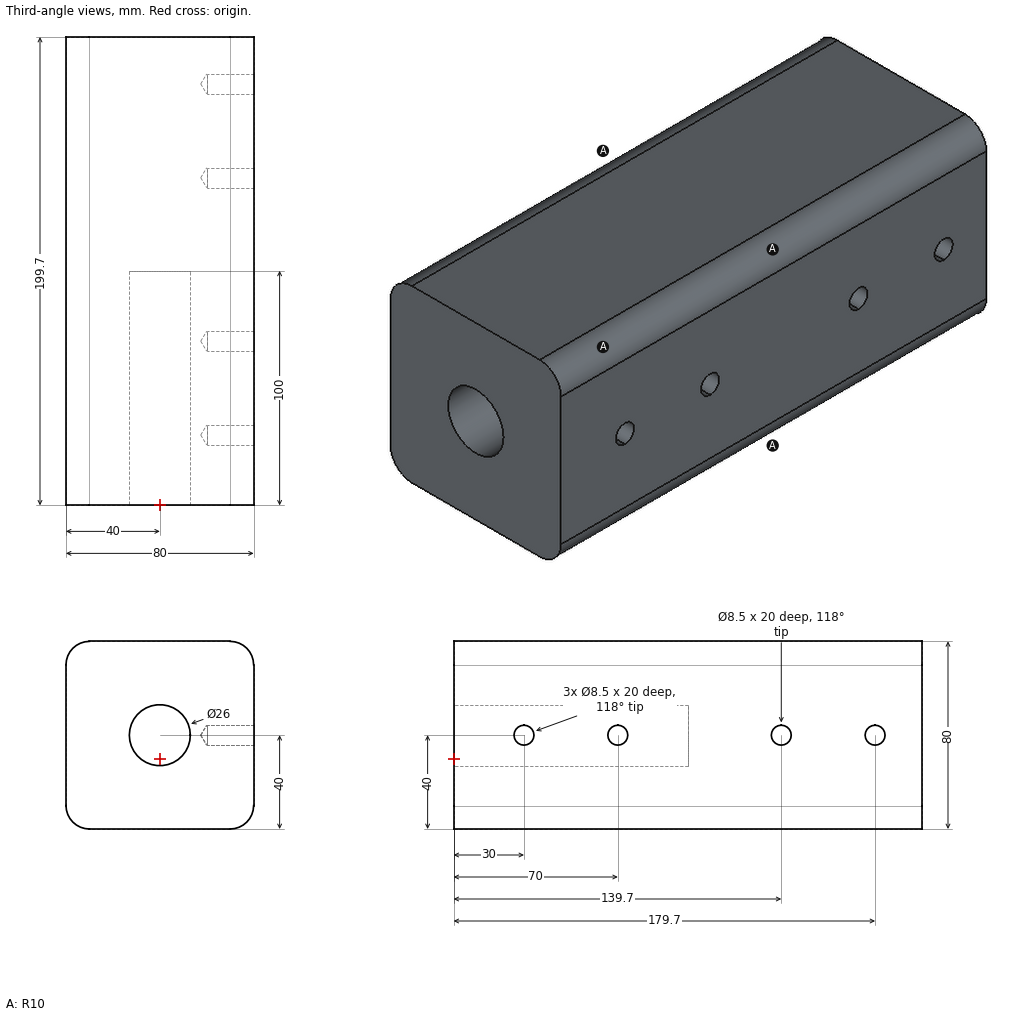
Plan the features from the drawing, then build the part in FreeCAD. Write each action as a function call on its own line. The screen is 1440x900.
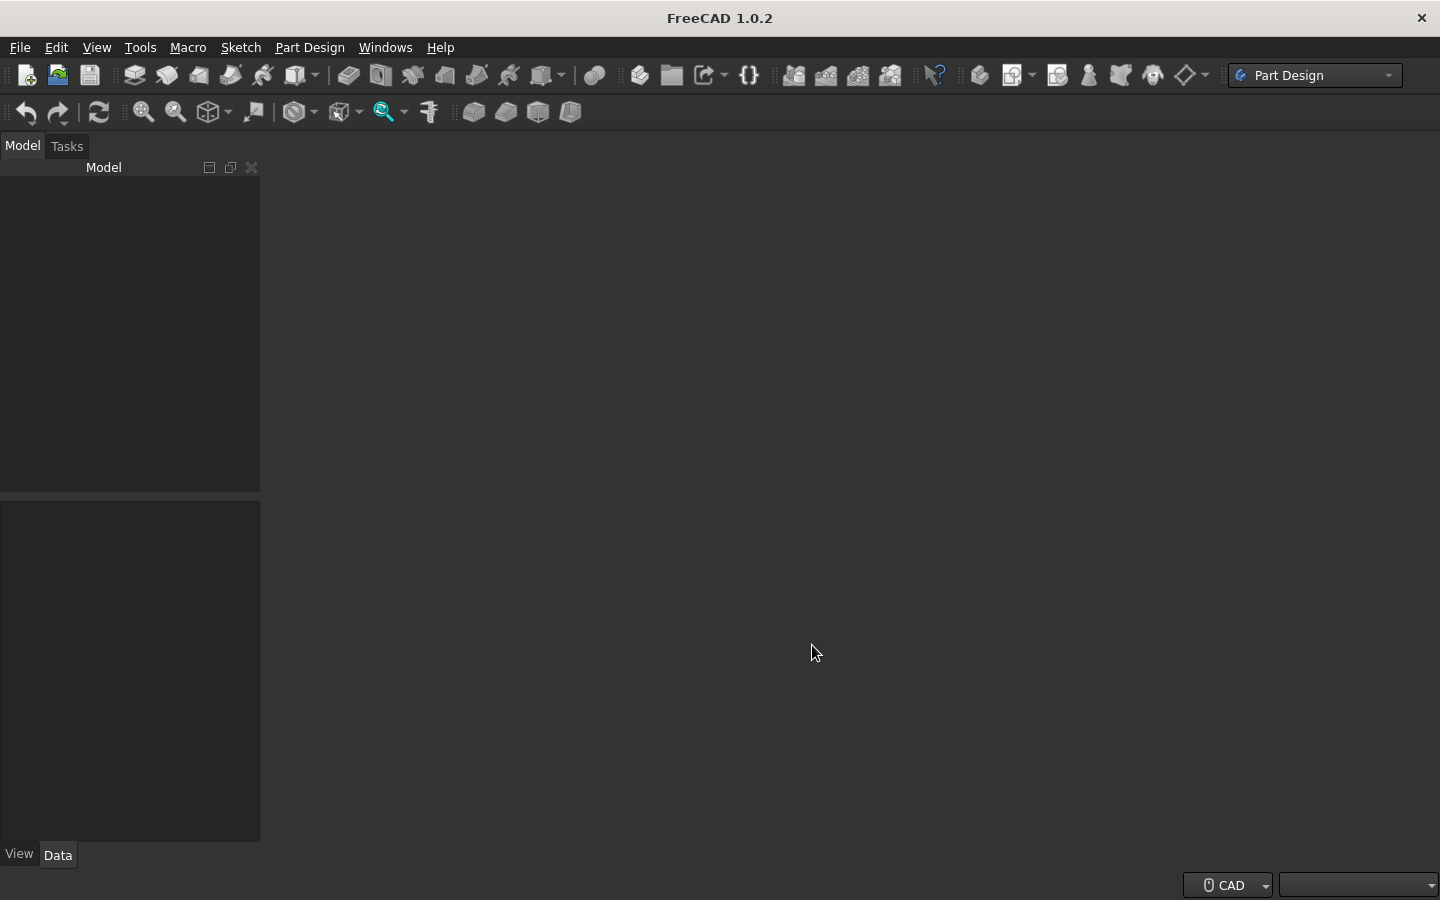
click(26, 76)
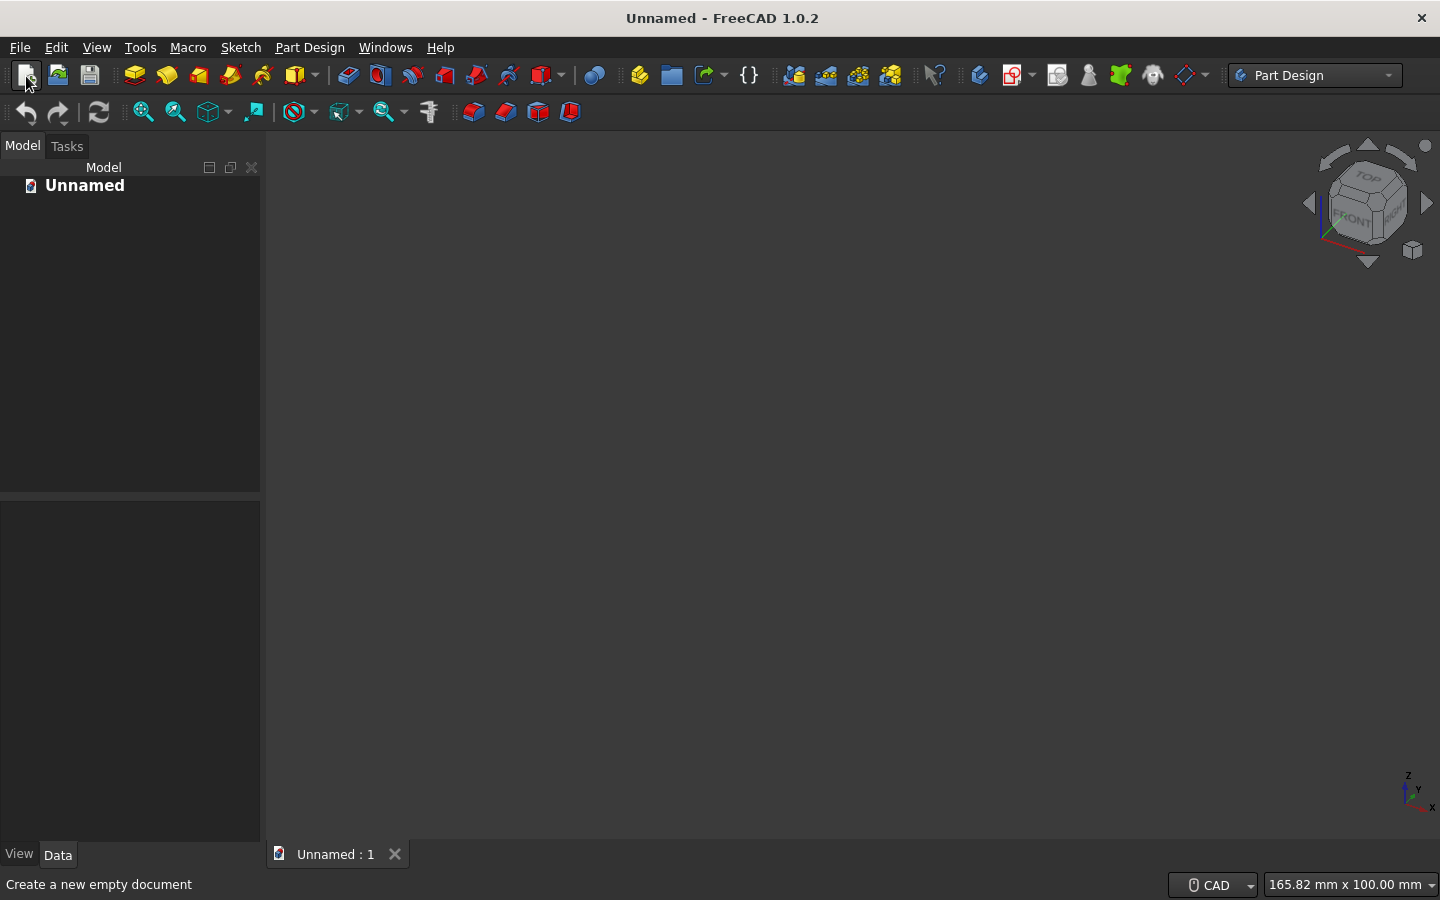
click(980, 76)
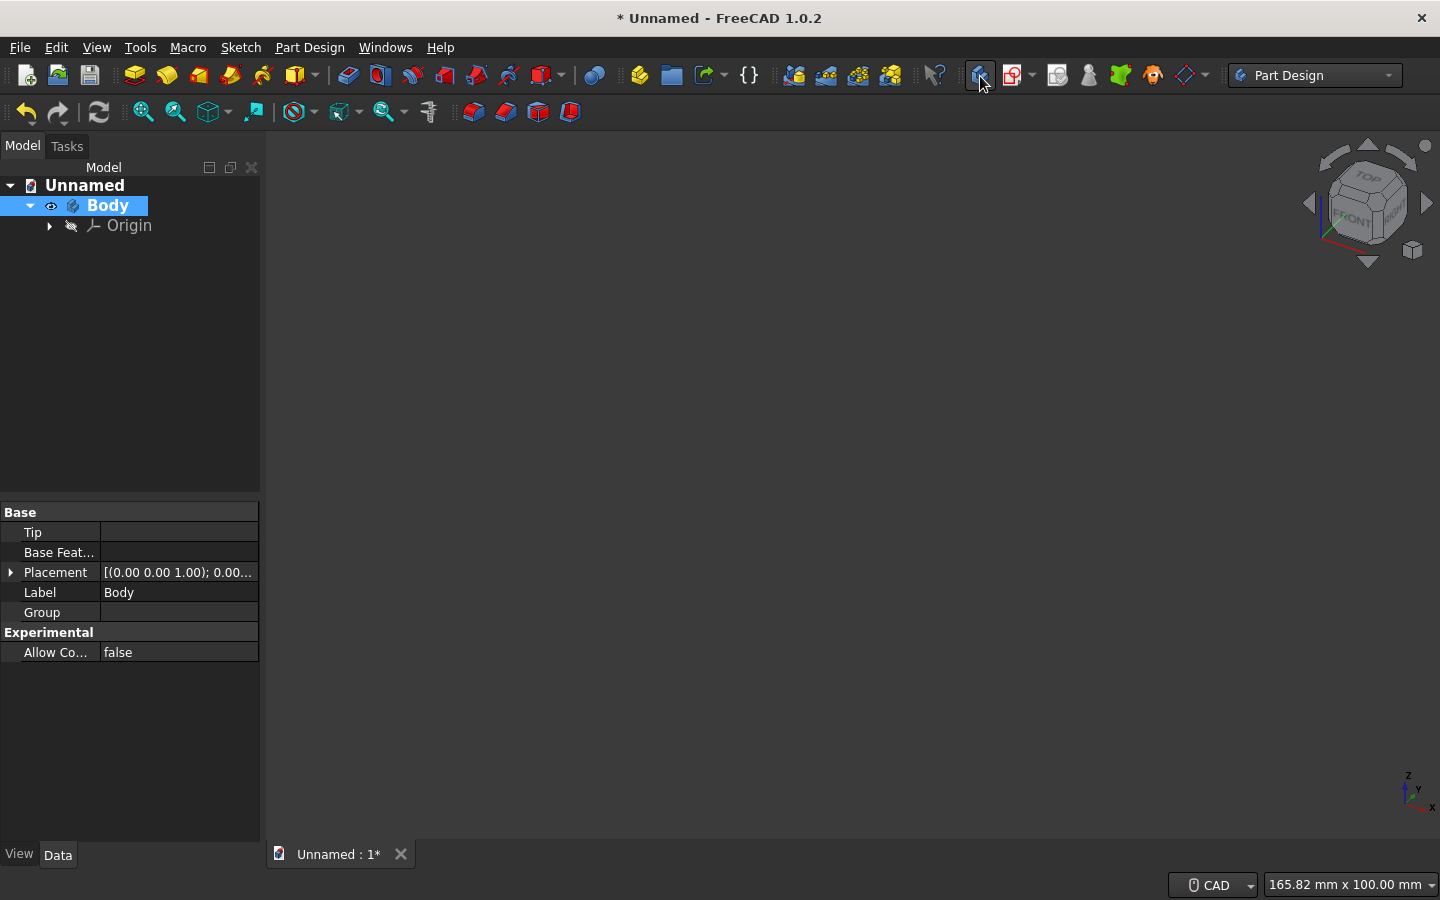
click(50, 226)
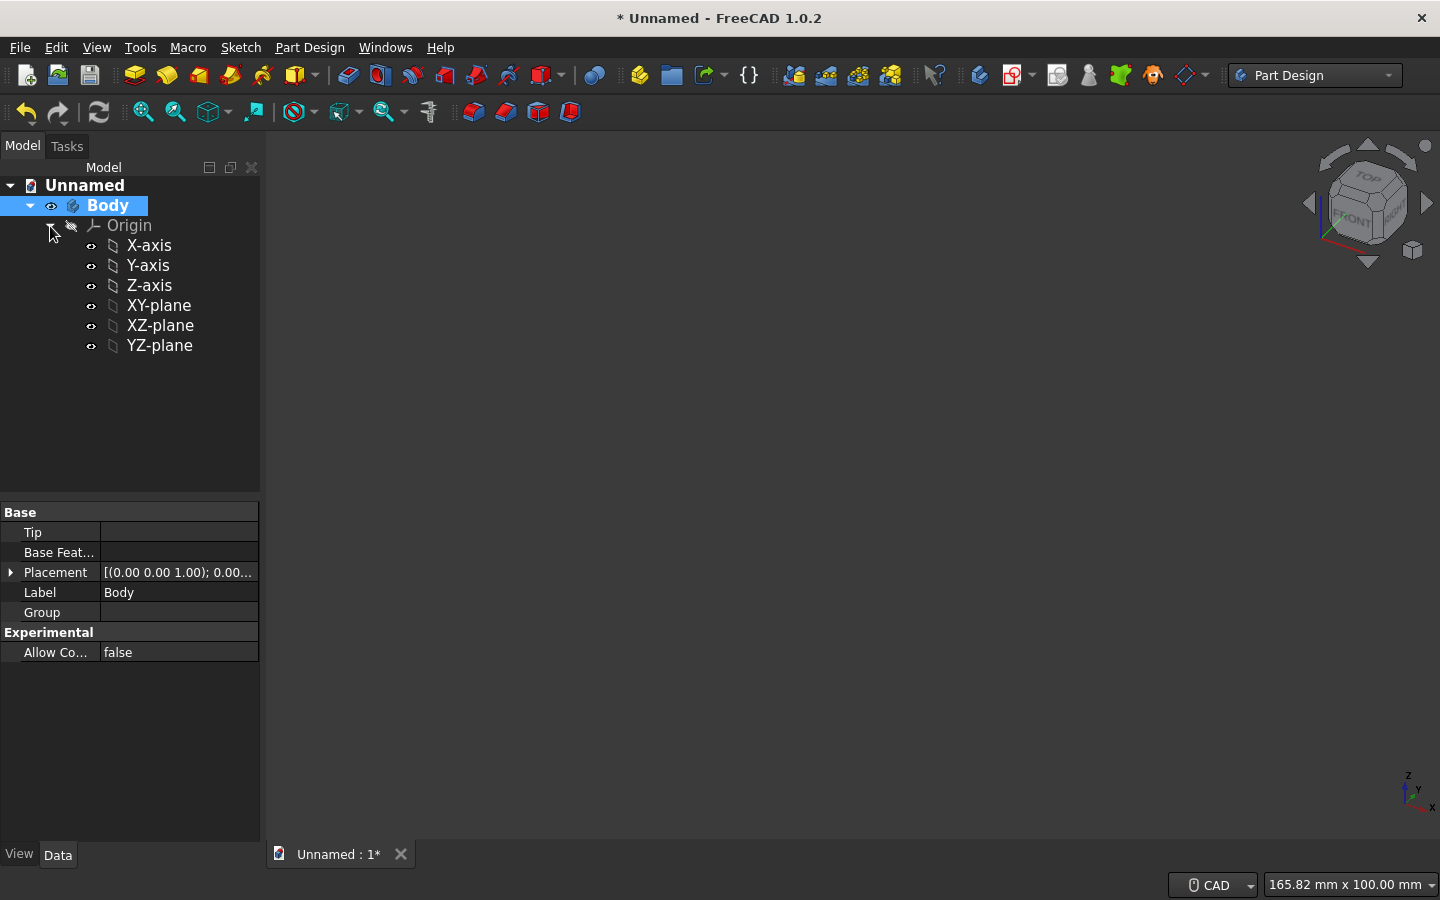
click(136, 306)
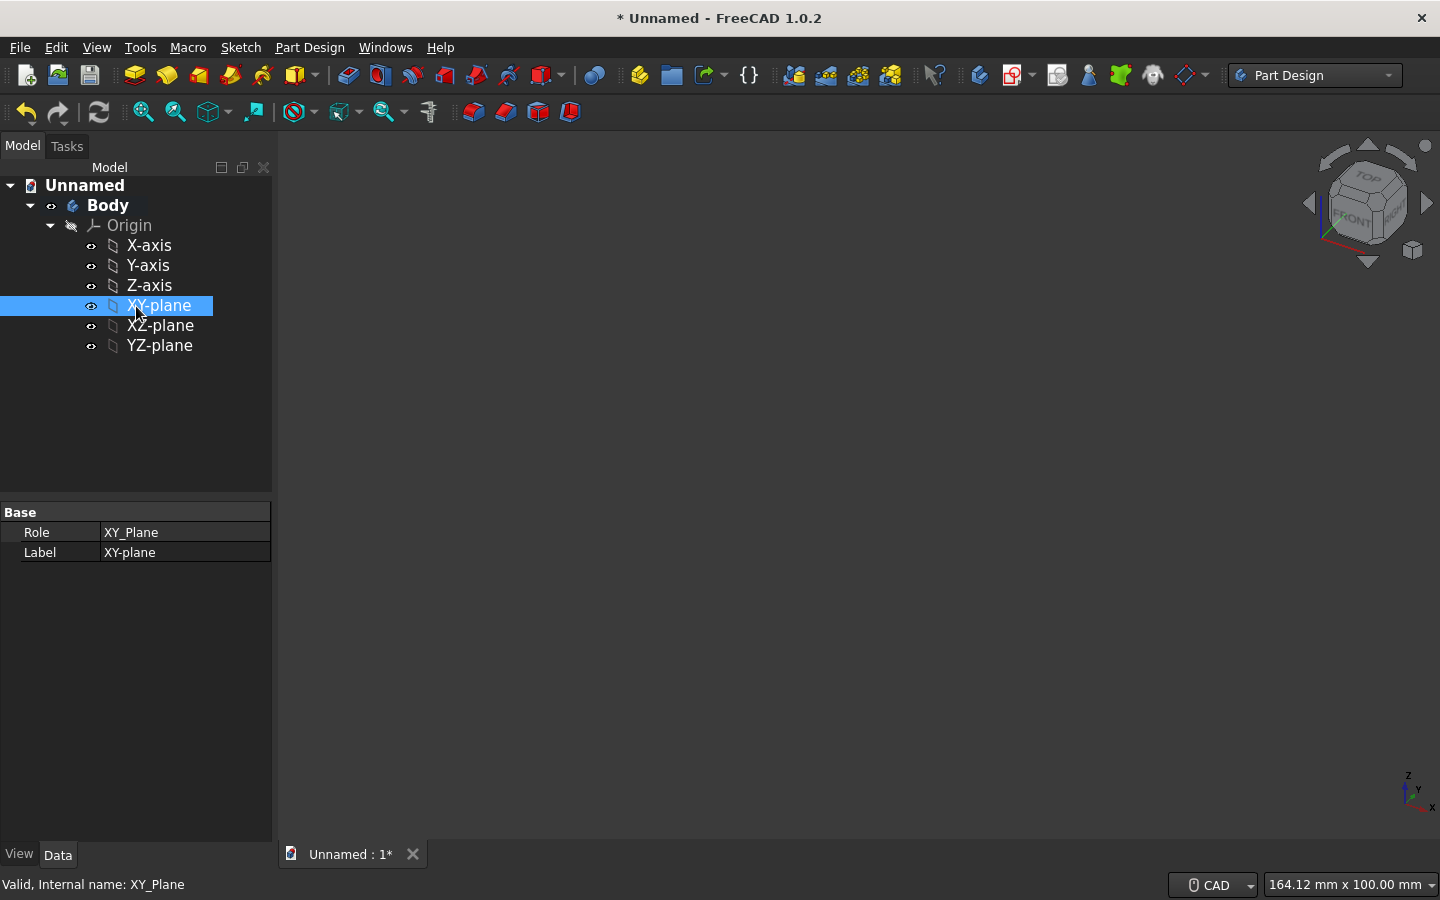
click(1186, 76)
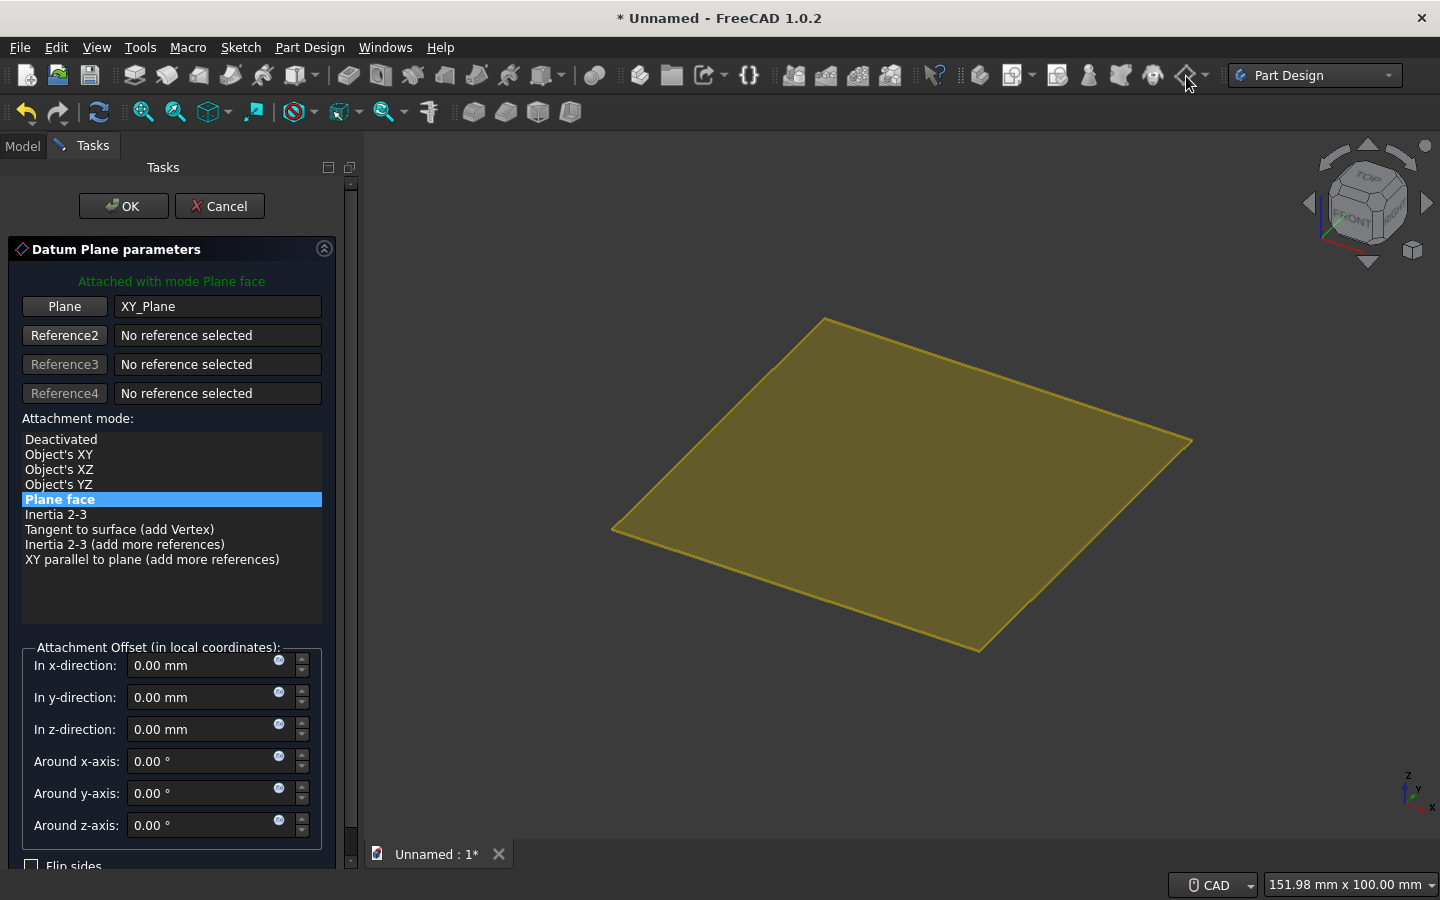
triple_click(210, 729)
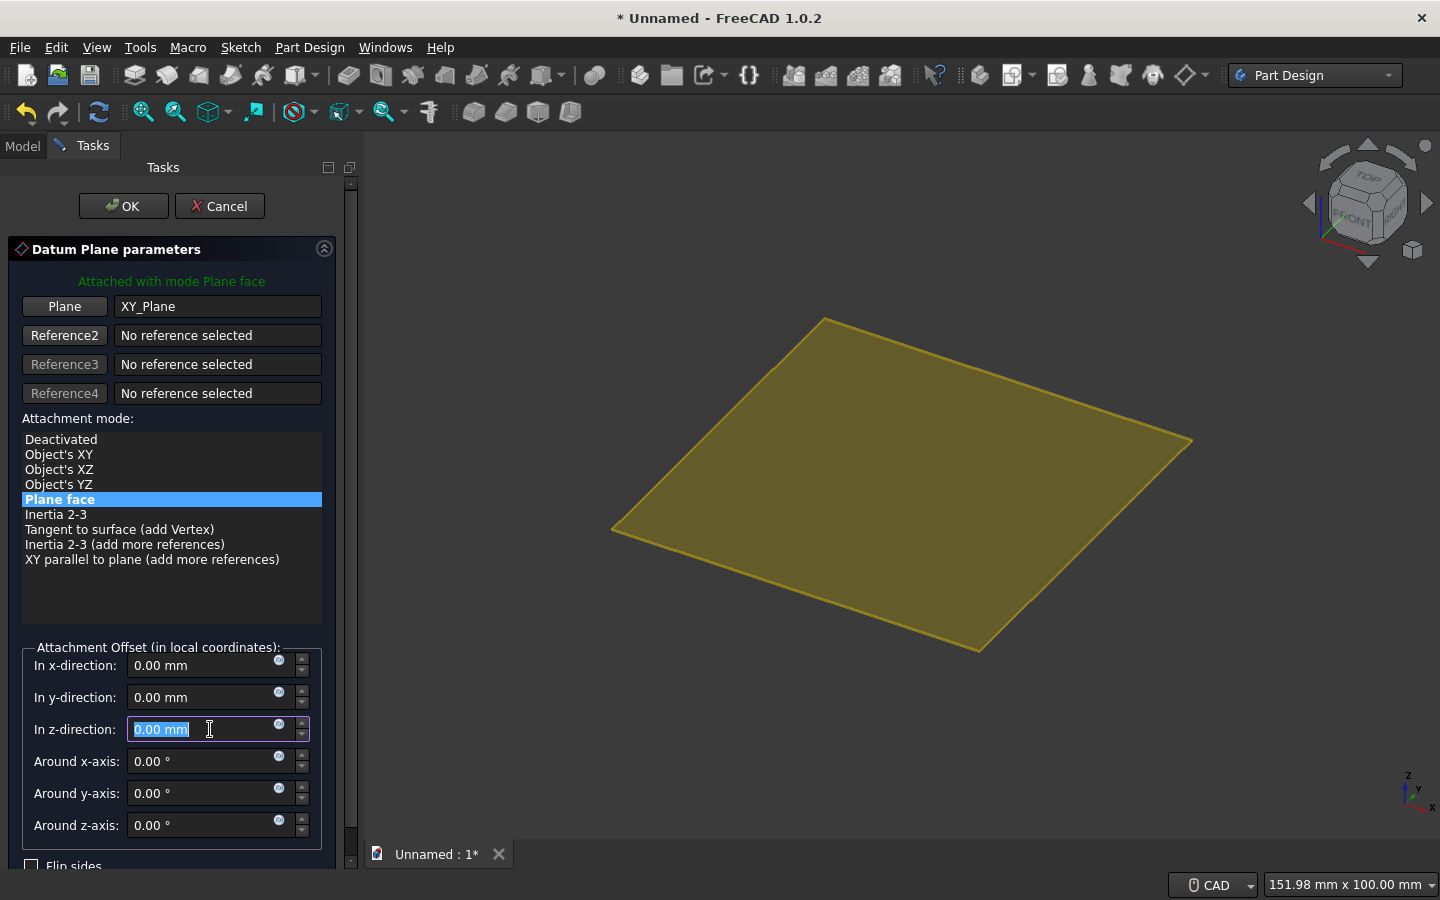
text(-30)
key(Tab)